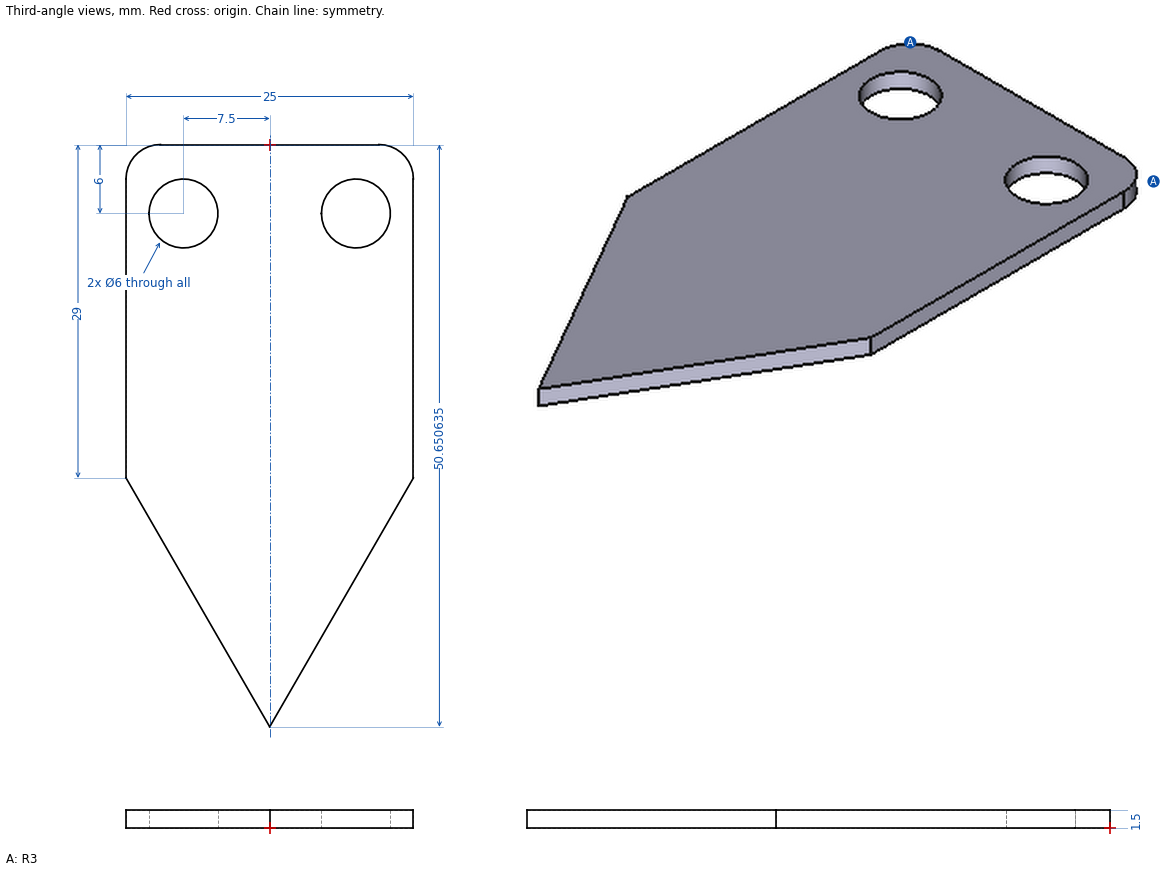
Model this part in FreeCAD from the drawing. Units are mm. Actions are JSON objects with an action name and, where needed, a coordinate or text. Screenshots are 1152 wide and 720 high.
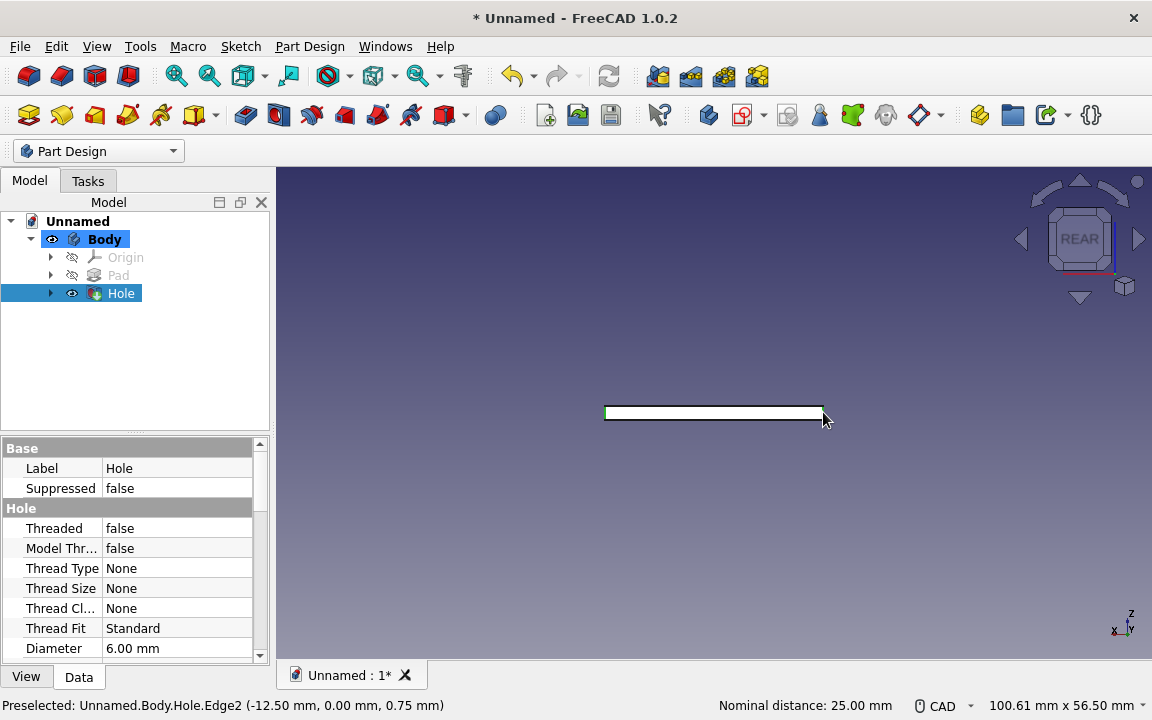
{"action": "left_click", "coordinate": [29, 76]}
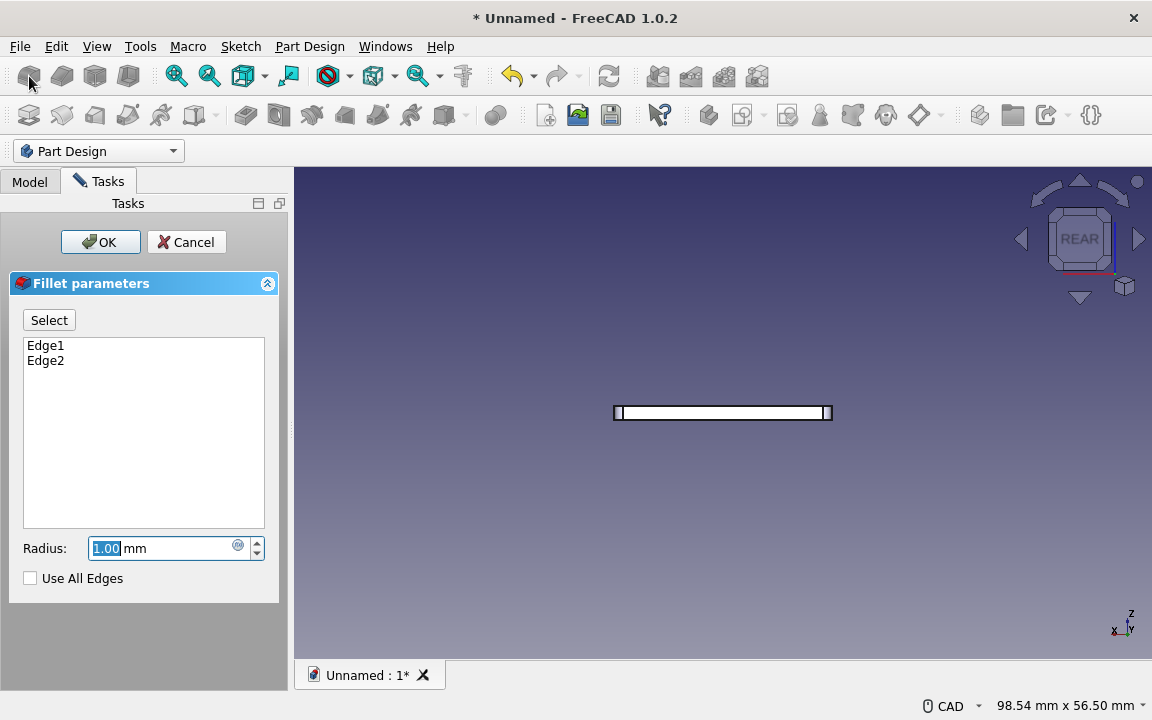
{"action": "type", "text": "3"}
{"action": "key", "text": "Tab"}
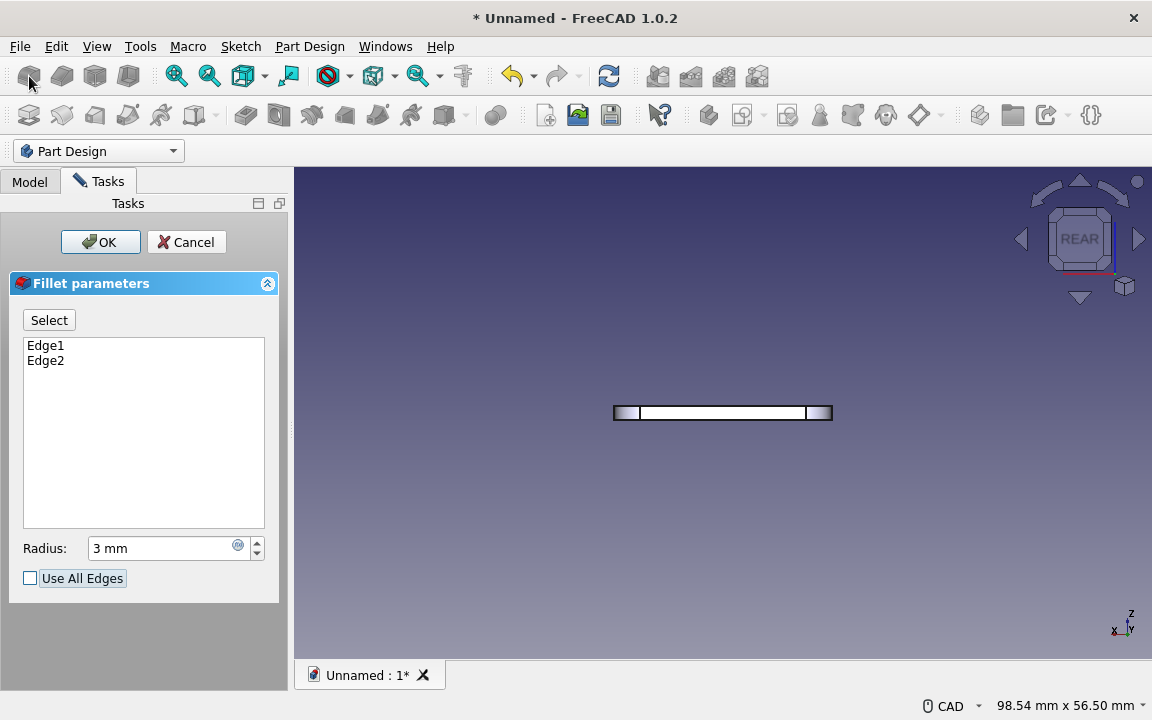
{"action": "left_click", "coordinate": [101, 242]}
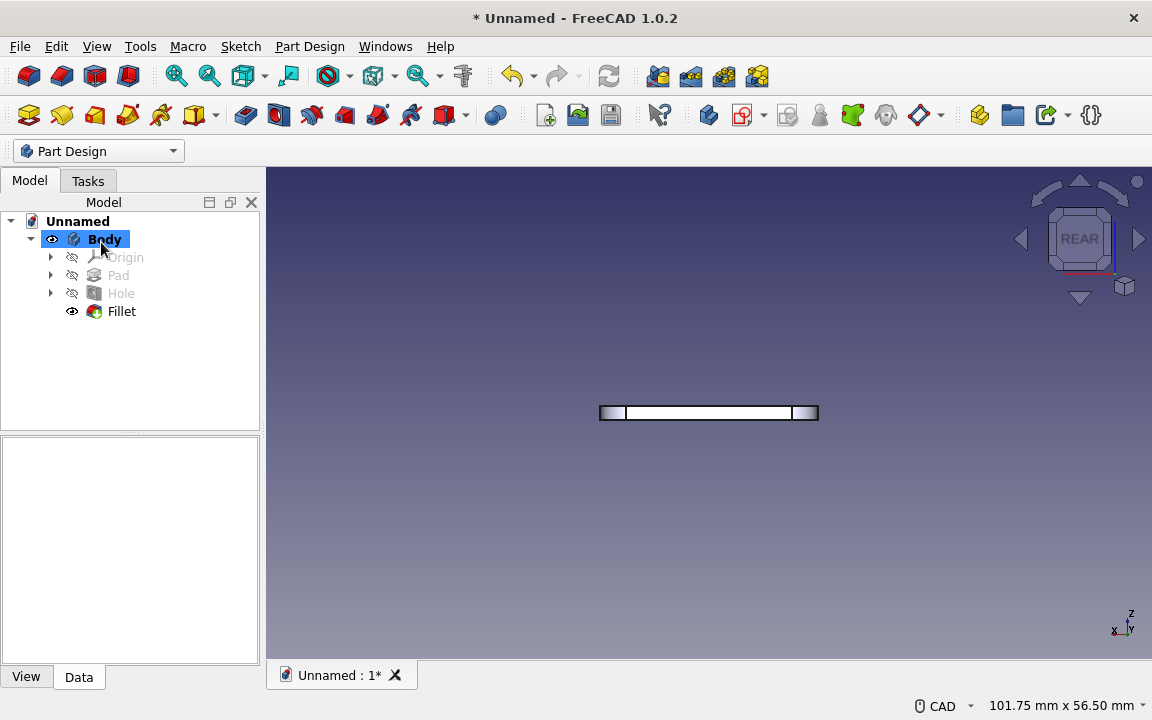
{"action": "key", "text": "0"}